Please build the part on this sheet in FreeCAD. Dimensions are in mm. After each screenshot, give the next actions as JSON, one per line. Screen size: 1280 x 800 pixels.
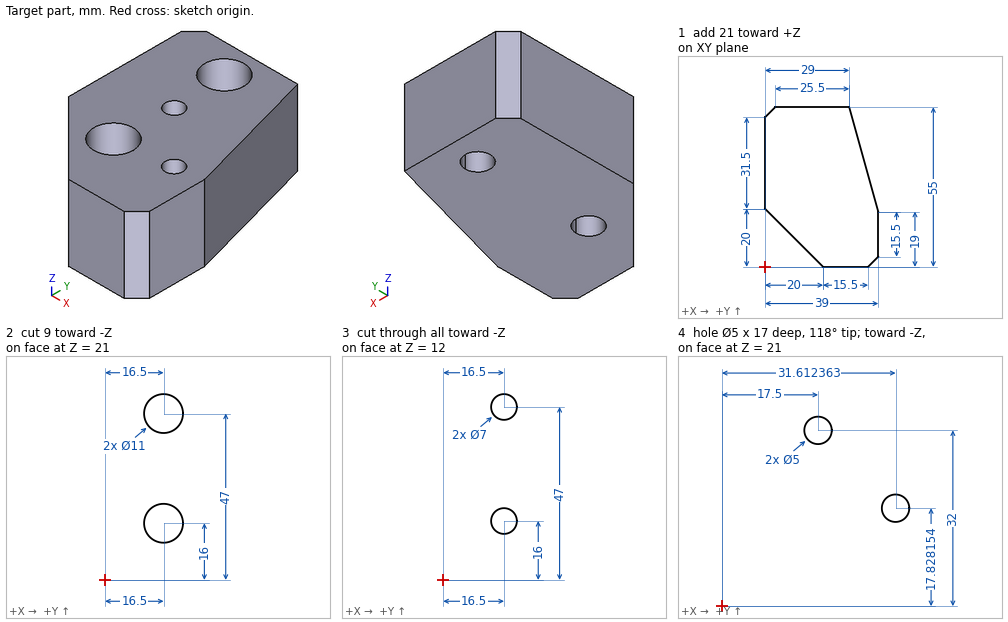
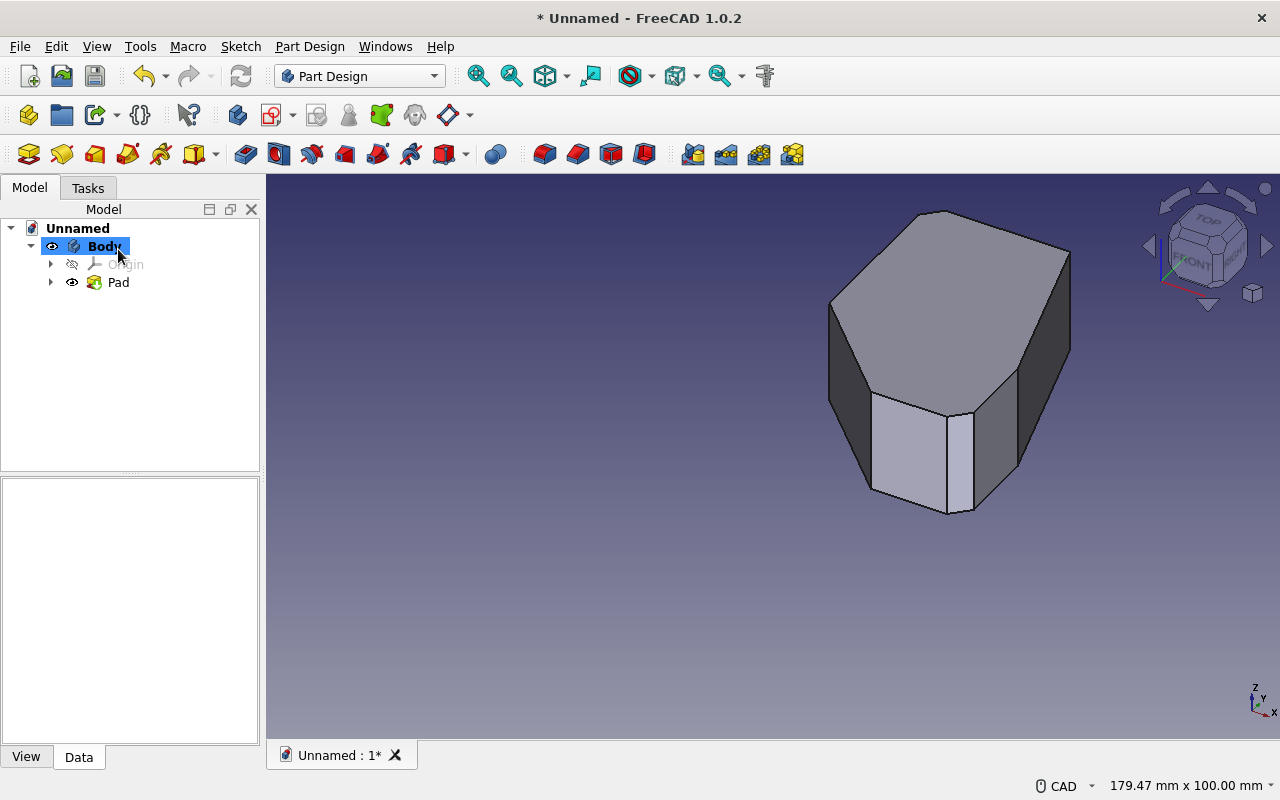
{"action": "left_click", "coordinate": [946, 313]}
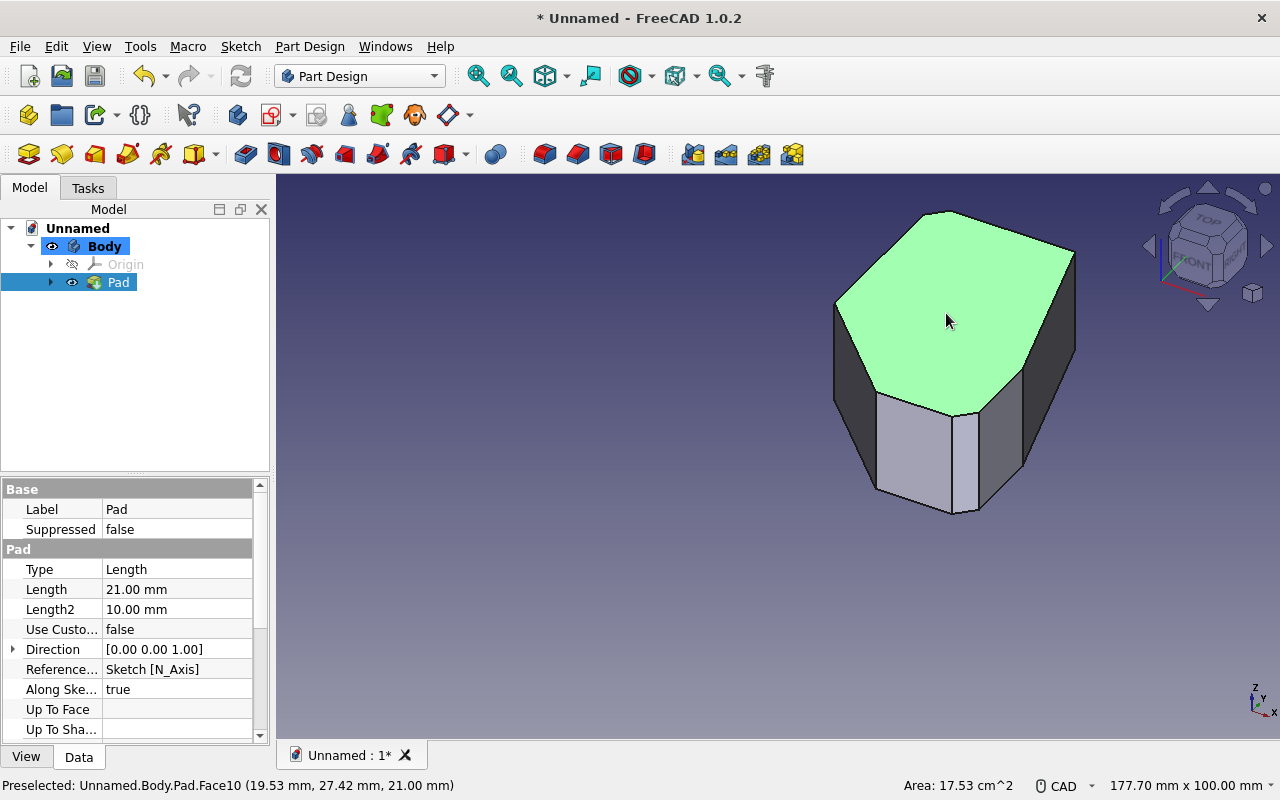
{"action": "left_click", "coordinate": [270, 116]}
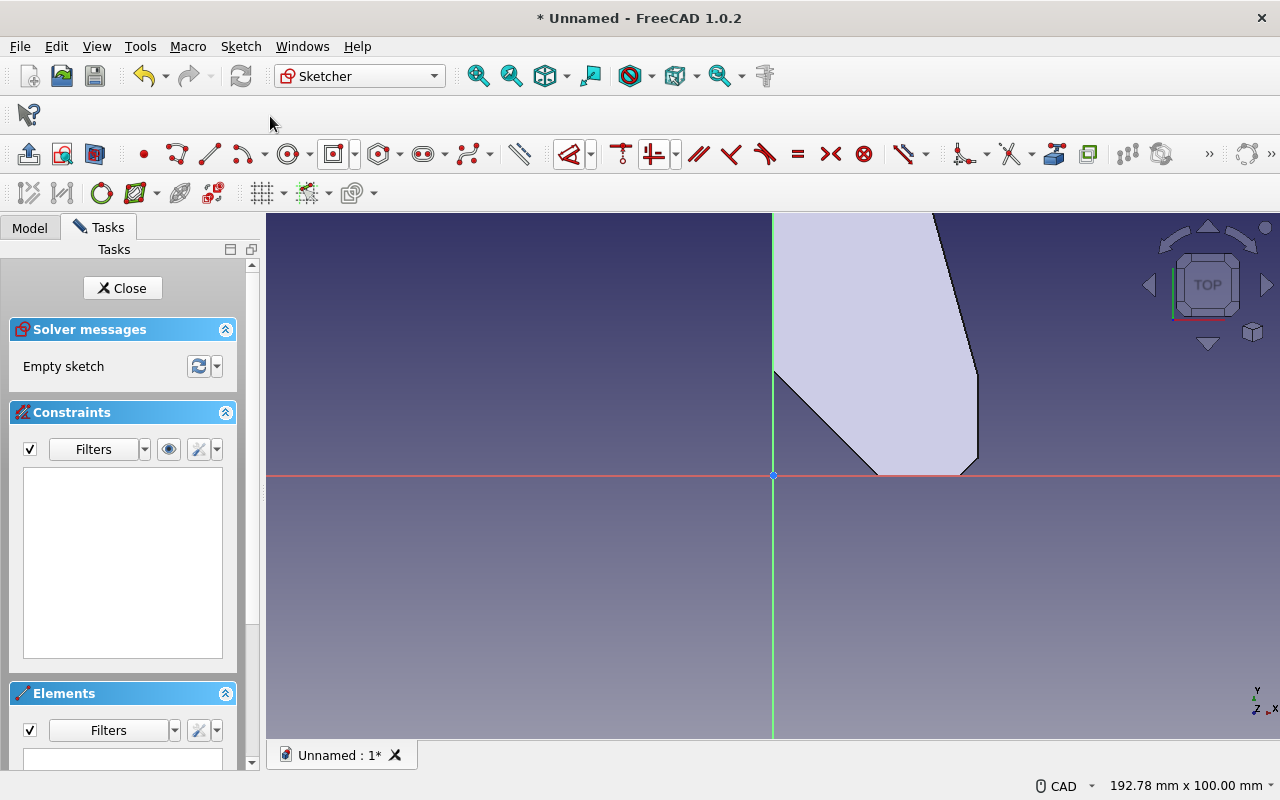
{"action": "scroll", "coordinate": [294, 711], "scroll_direction": "down", "scroll_amount": 1}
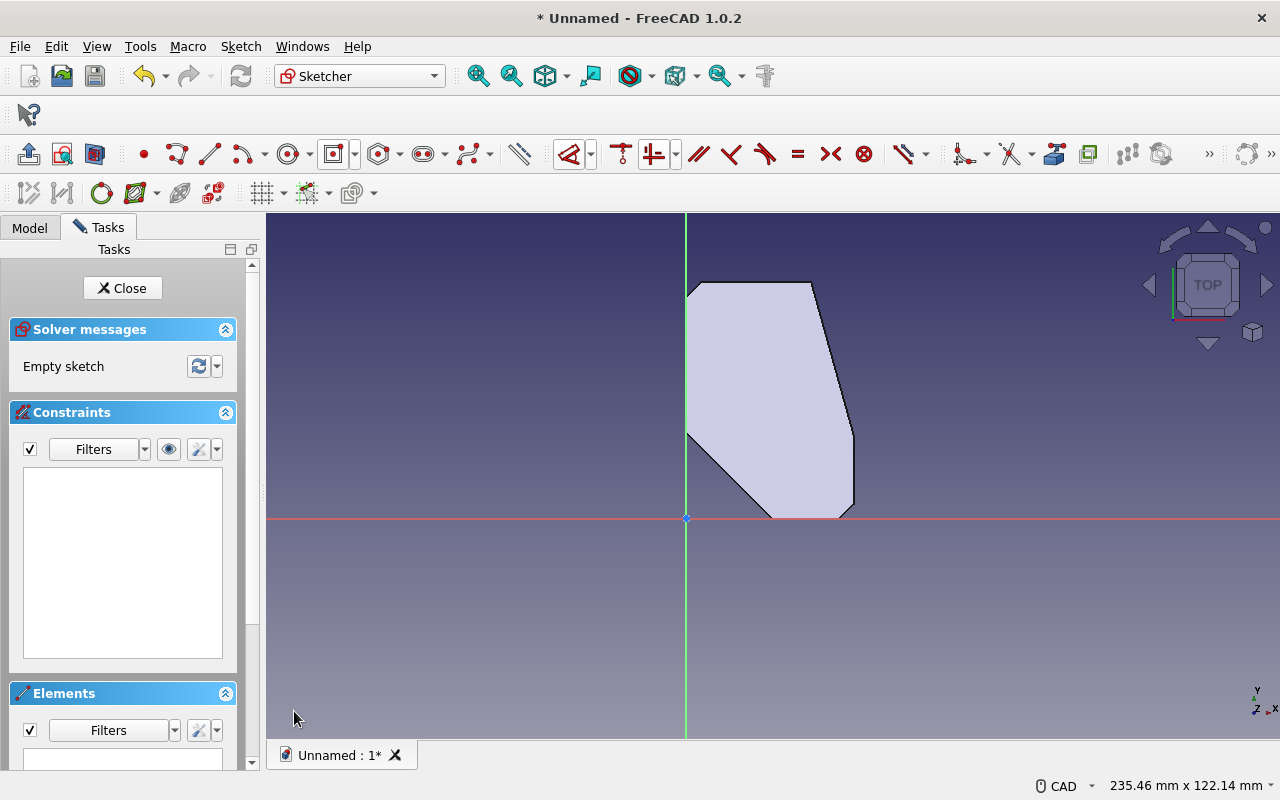
{"action": "scroll", "coordinate": [793, 263], "scroll_direction": "up", "scroll_amount": 2}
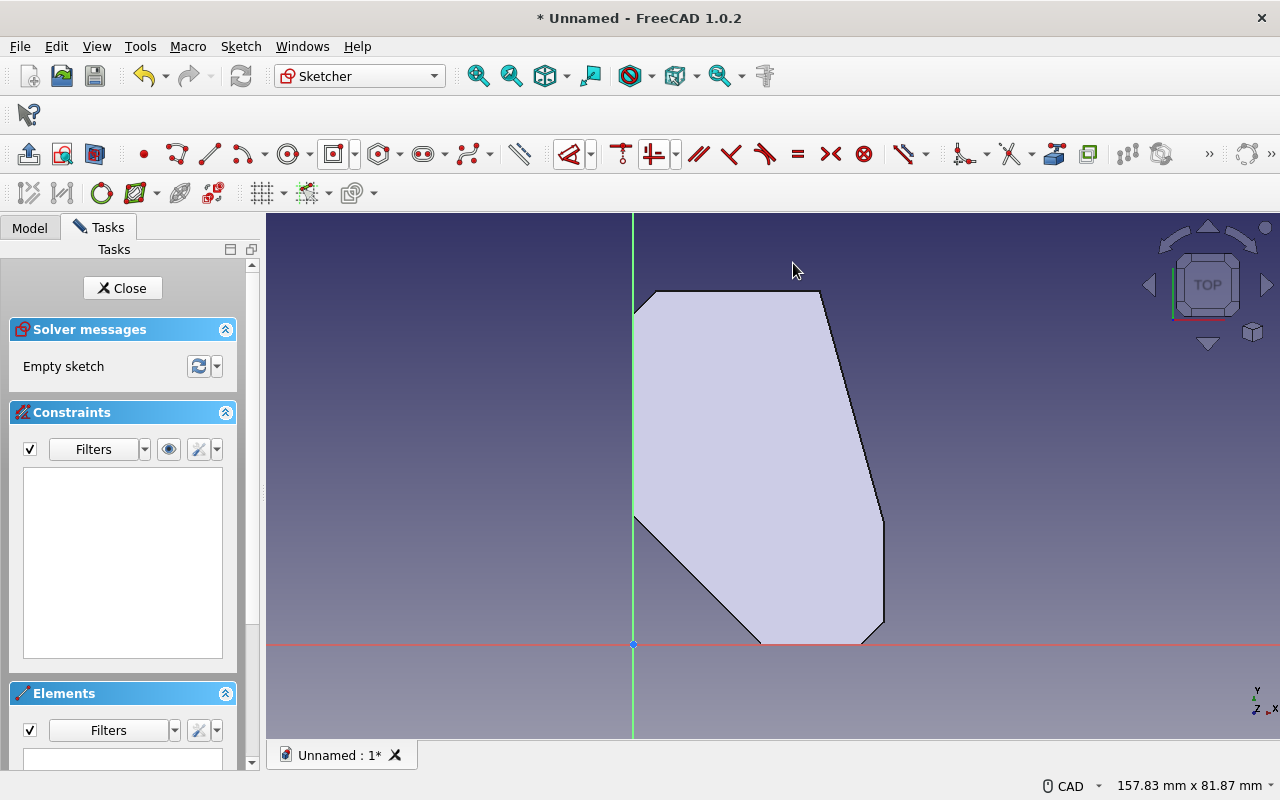
{"action": "left_click", "coordinate": [288, 154]}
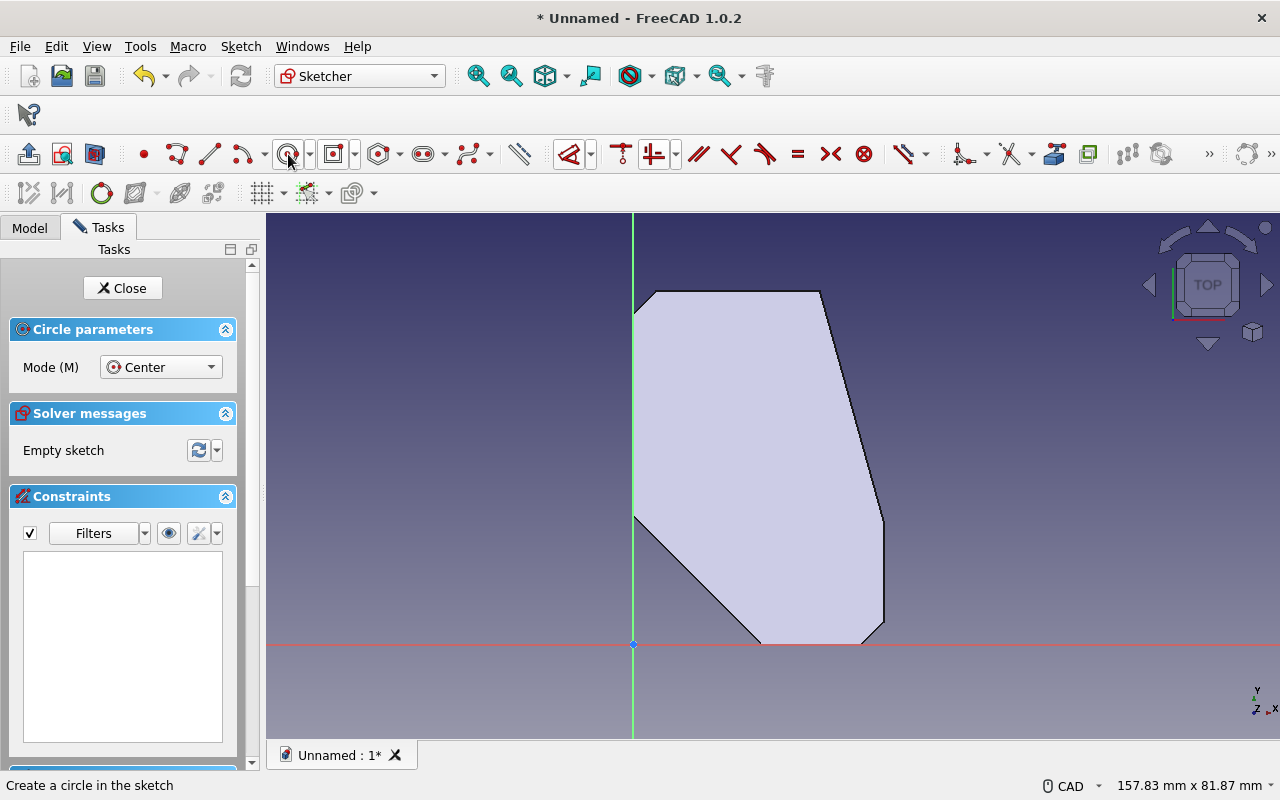
{"action": "left_click", "coordinate": [739, 343]}
{"action": "left_click", "coordinate": [764, 318]}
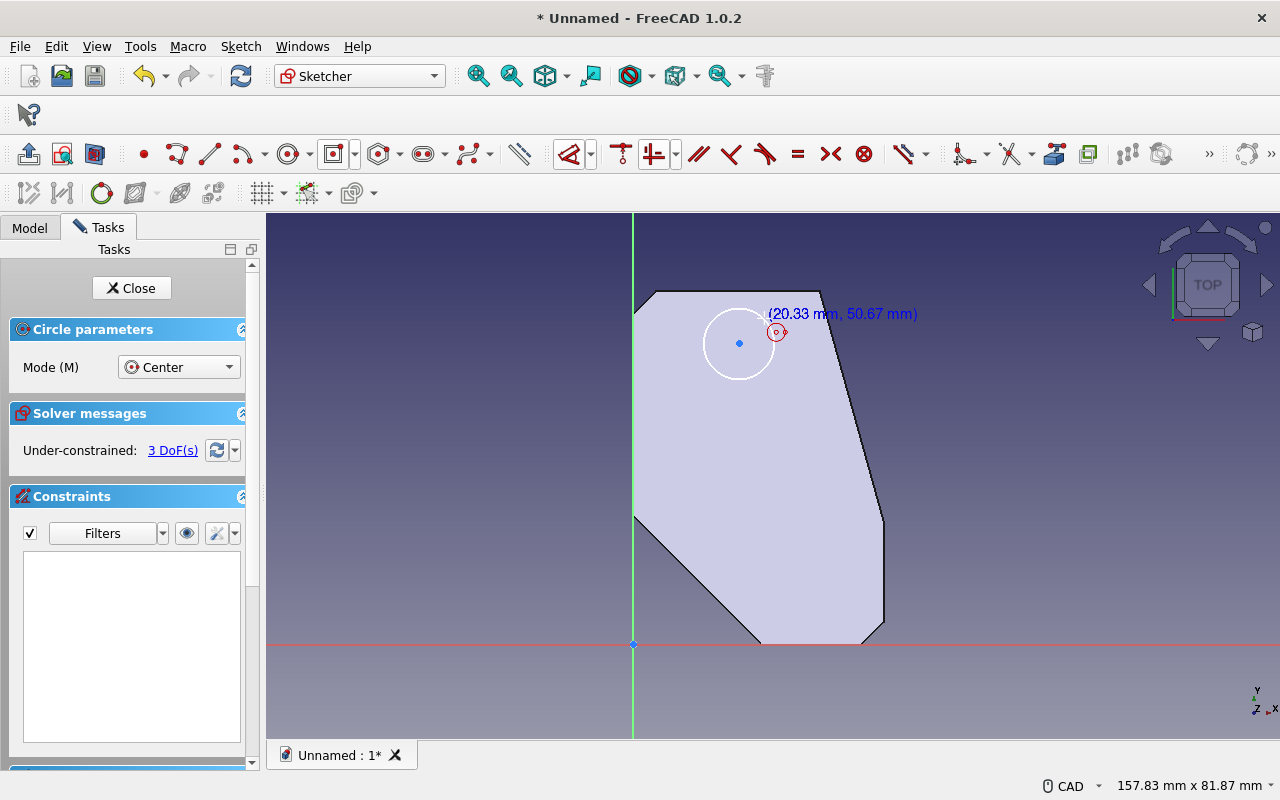
{"action": "left_click", "coordinate": [739, 542]}
{"action": "left_click", "coordinate": [764, 517]}
{"action": "key", "text": "Escape"}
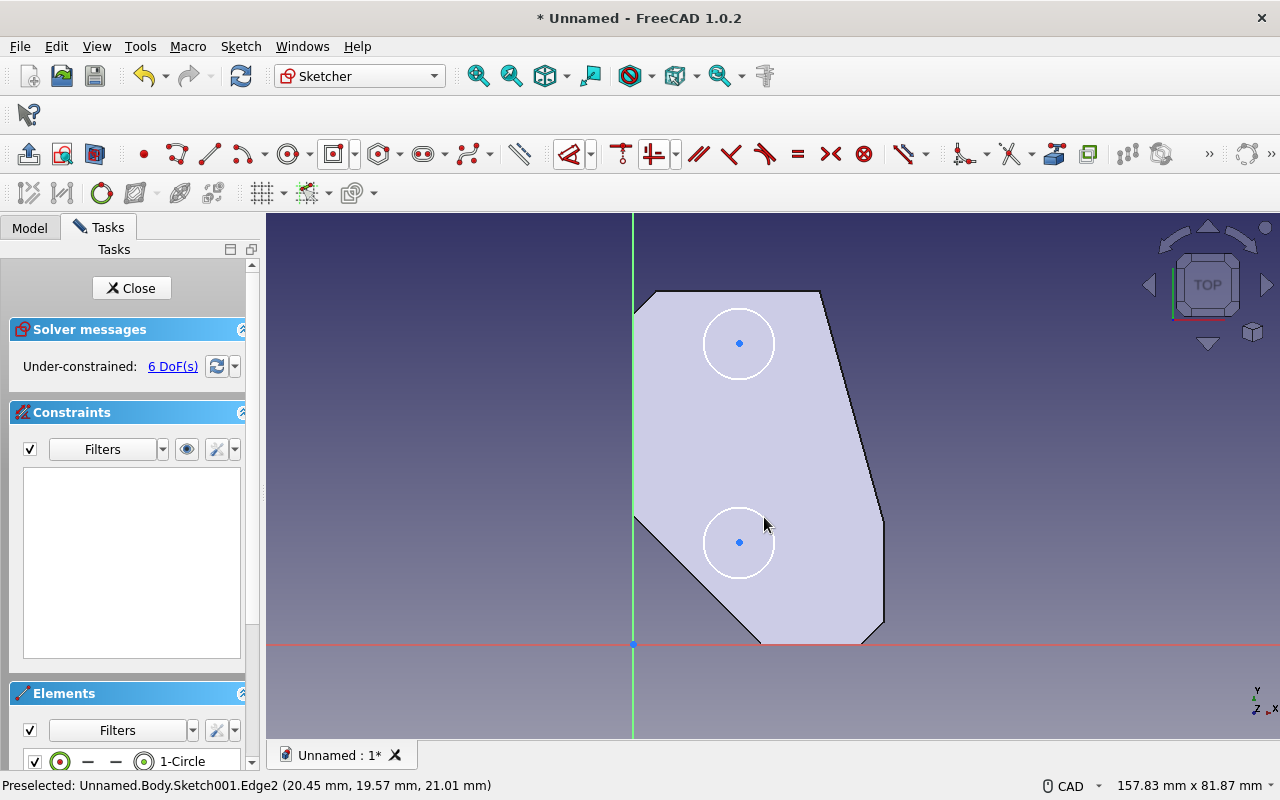
{"action": "left_click", "coordinate": [764, 319]}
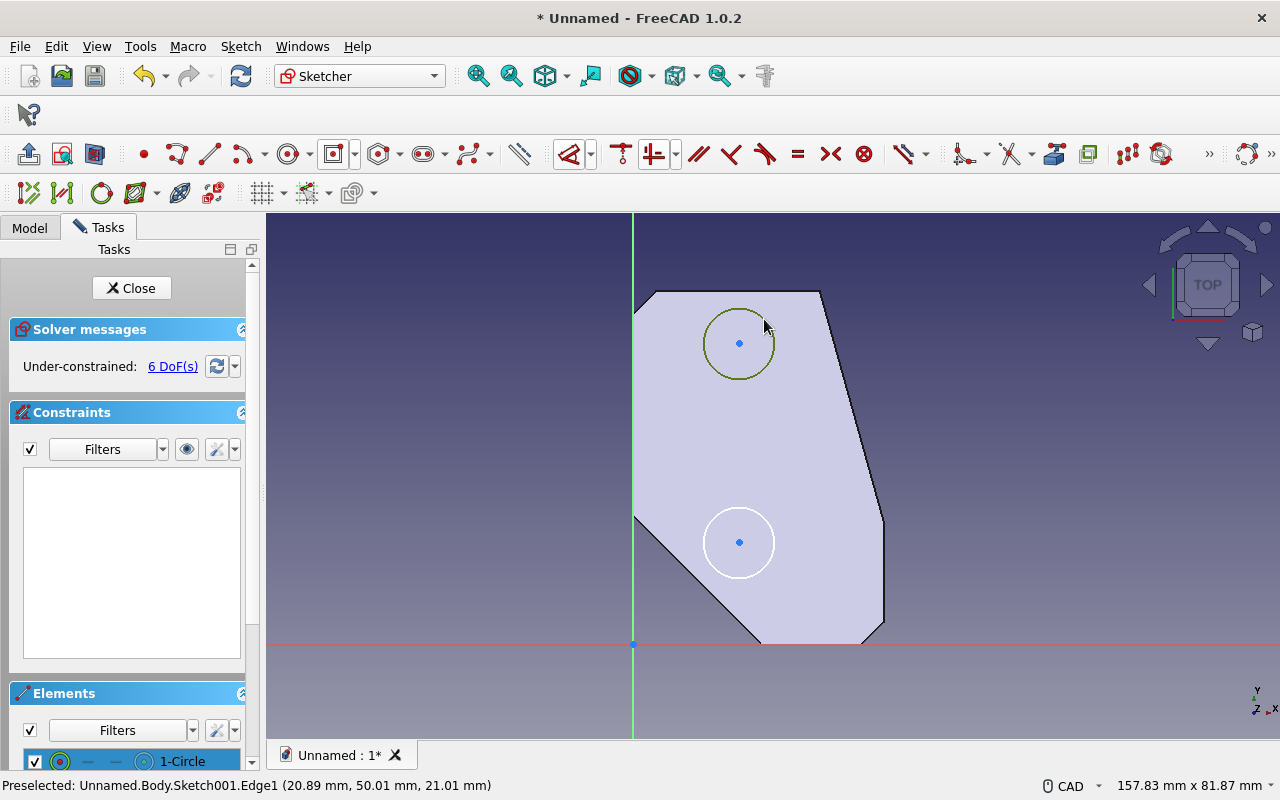
{"action": "left_click", "coordinate": [764, 518]}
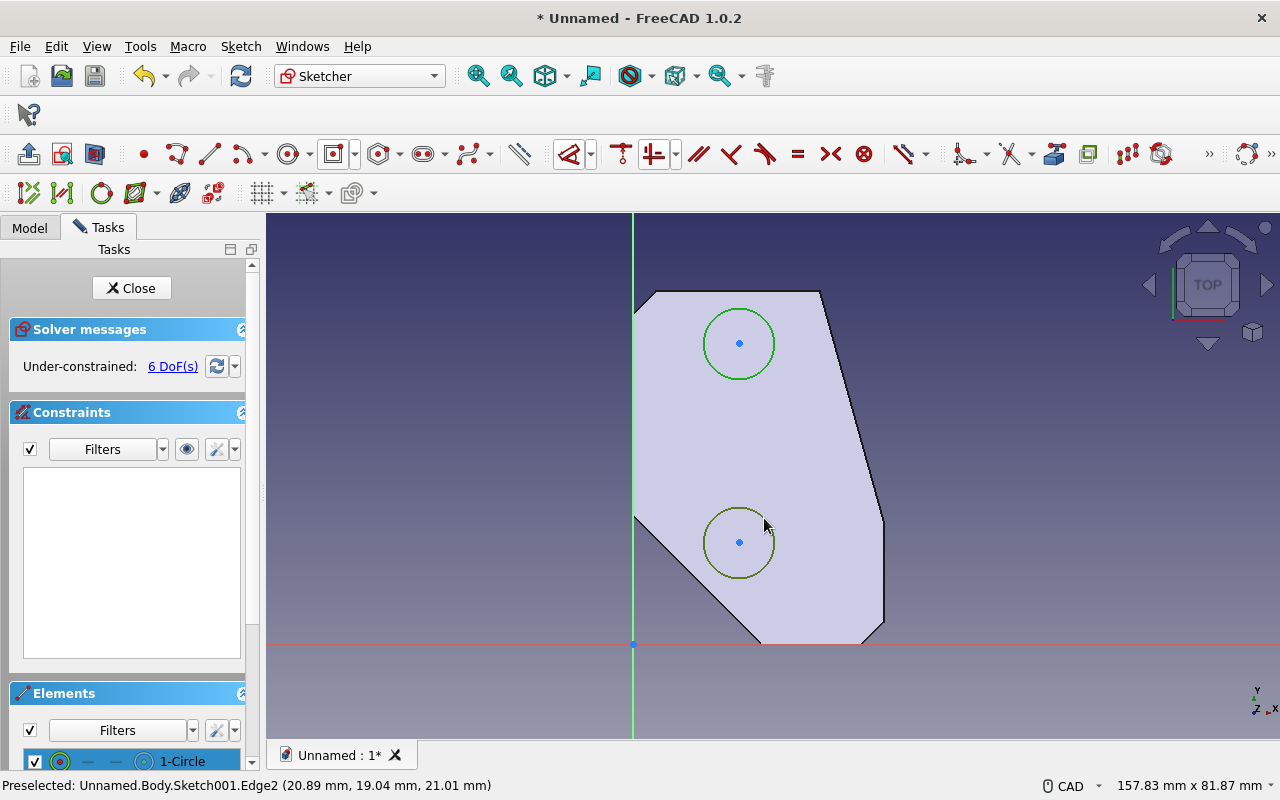
{"action": "left_click", "coordinate": [798, 154]}